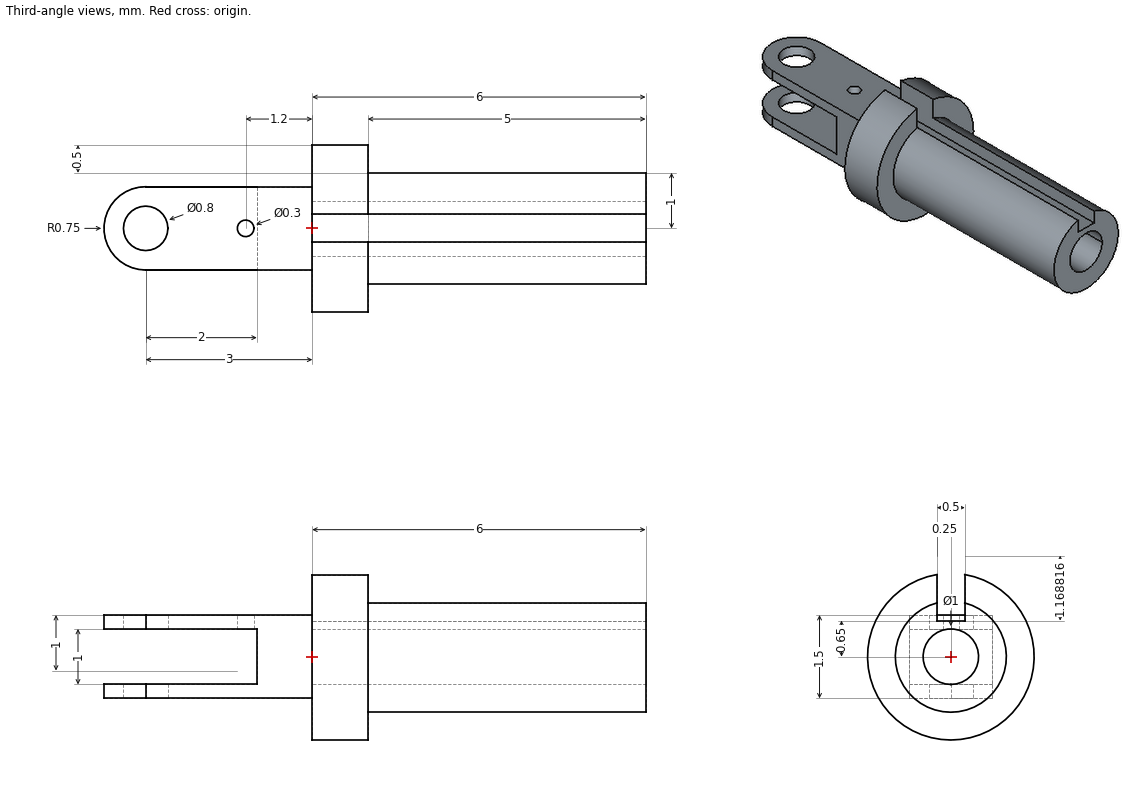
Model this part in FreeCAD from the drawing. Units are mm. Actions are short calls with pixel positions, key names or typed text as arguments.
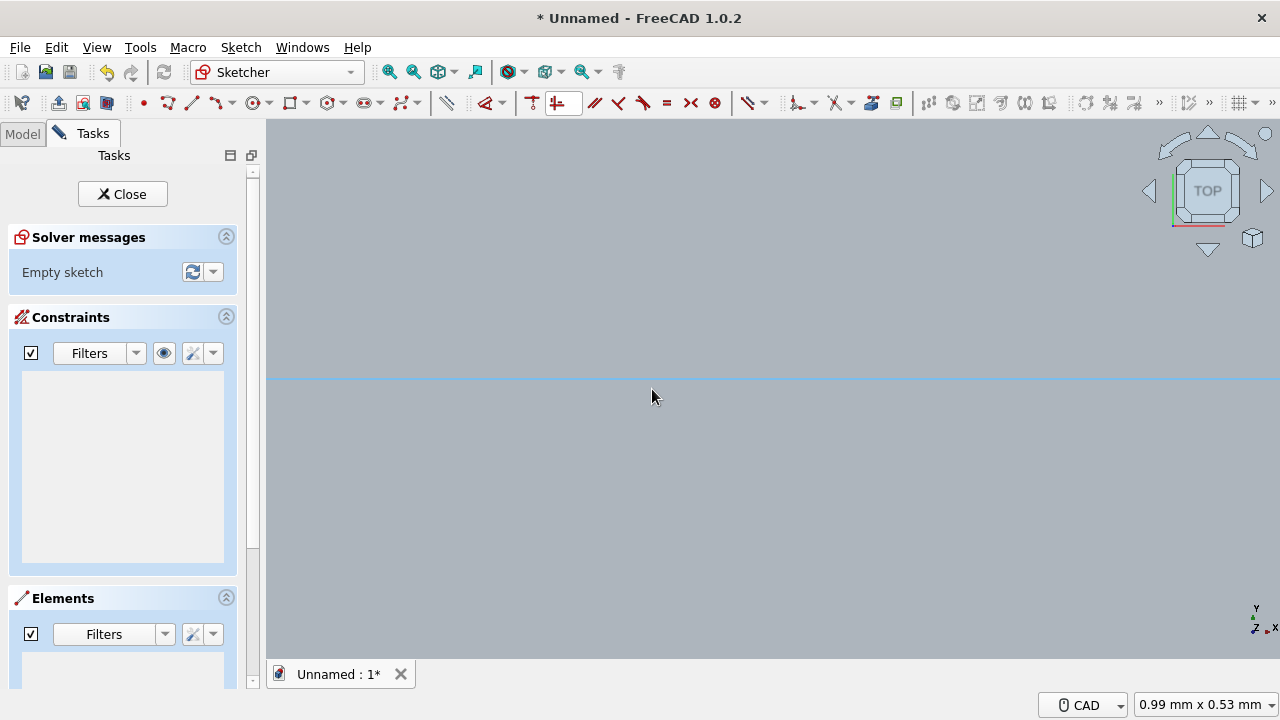
click(254, 104)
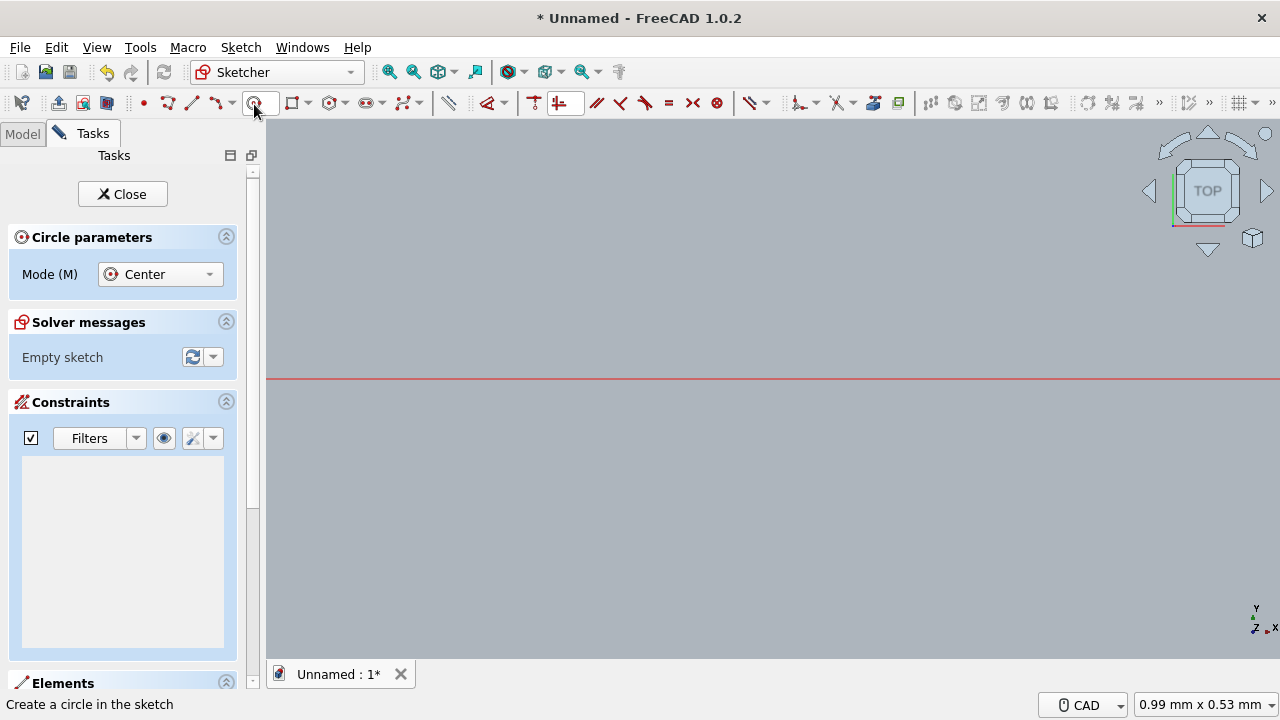
click(703, 379)
click(811, 271)
key(Escape)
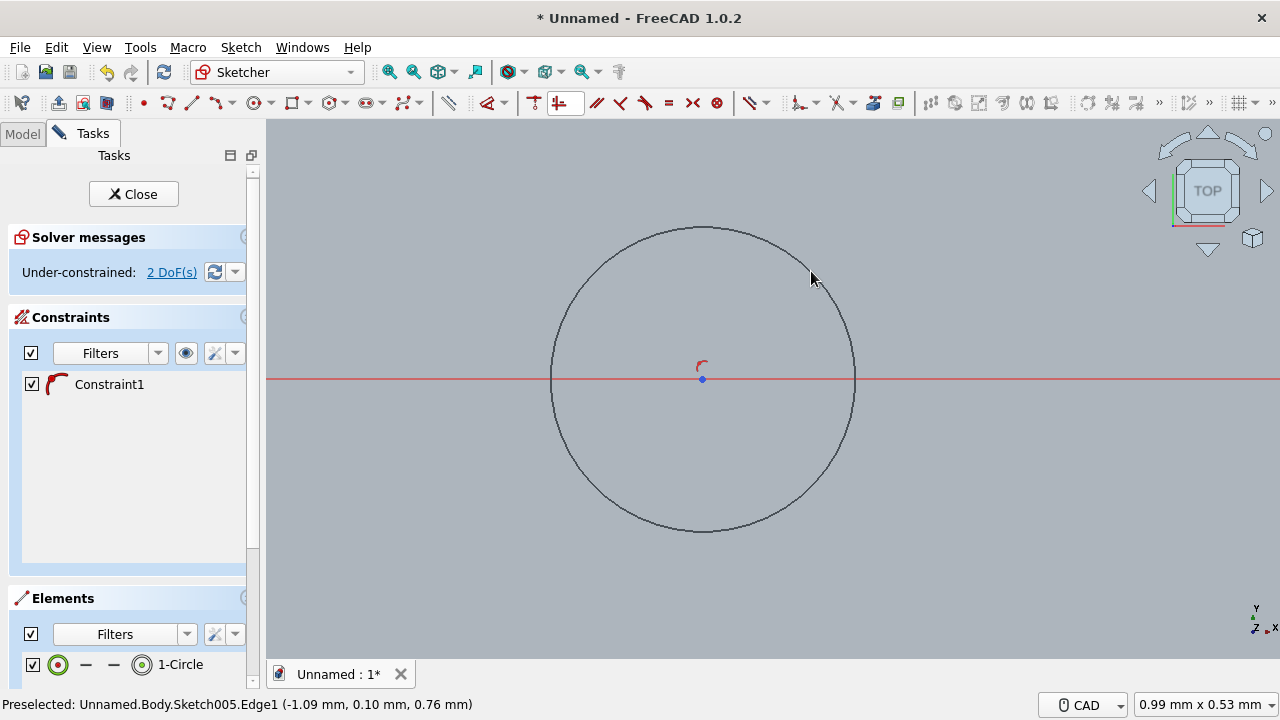
click(488, 104)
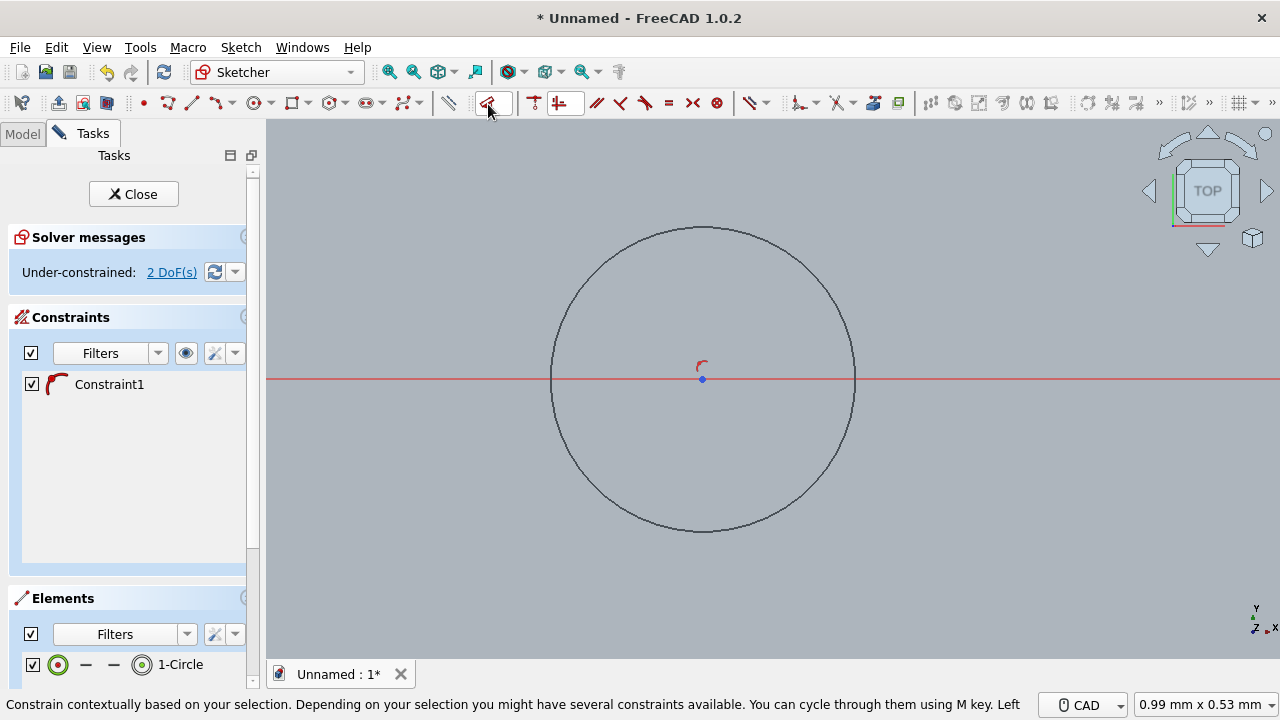
click(810, 271)
click(832, 248)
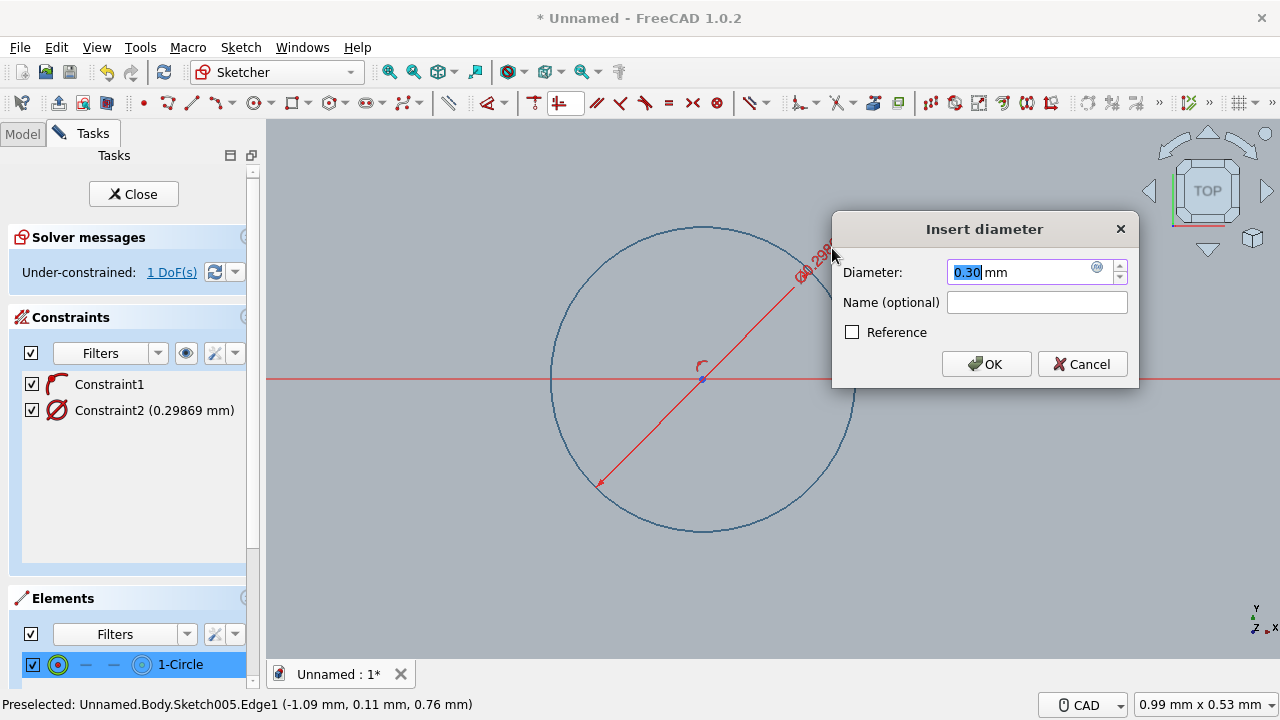
text(0.3)
key(Return)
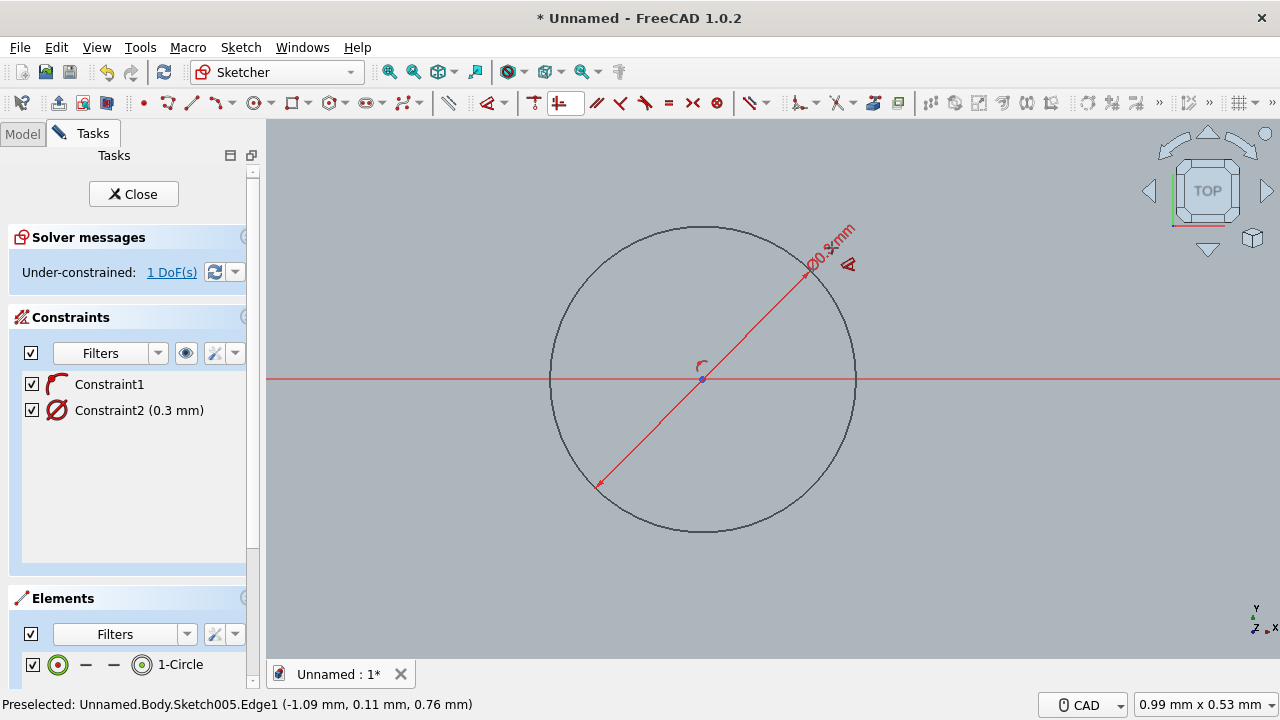
click(703, 379)
click(909, 413)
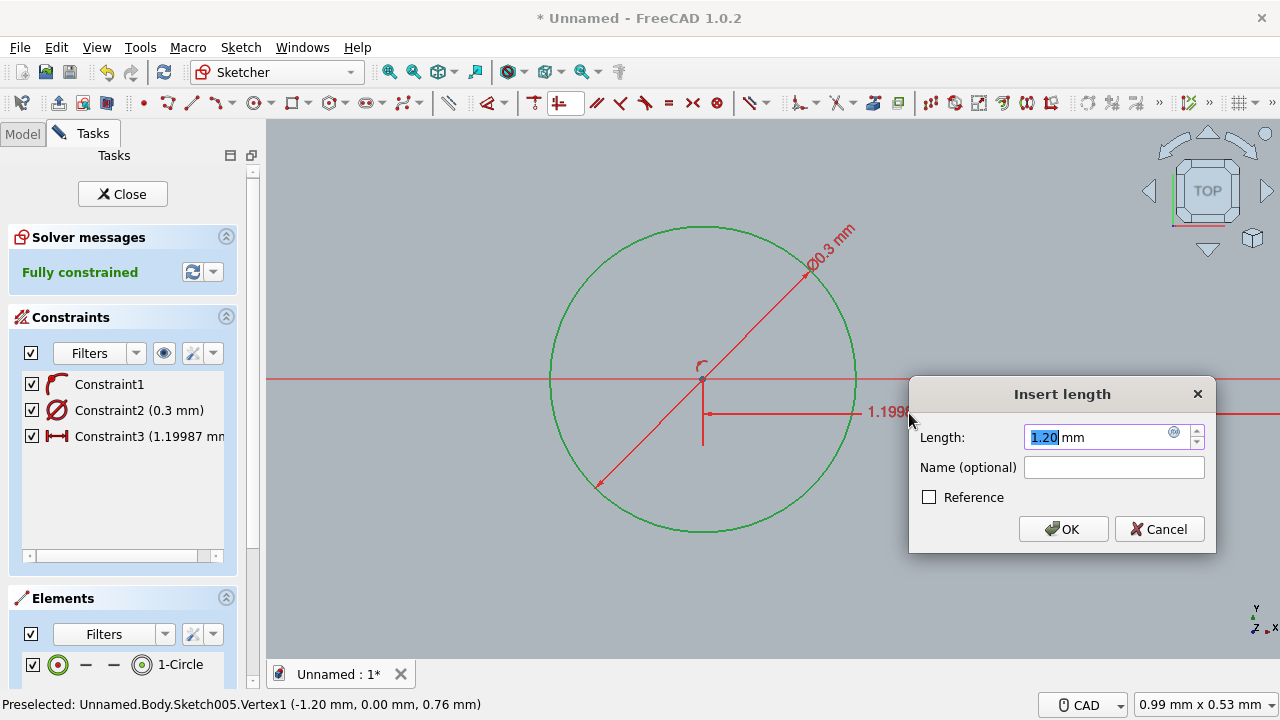
text(1.2)
key(Return)
key(Escape)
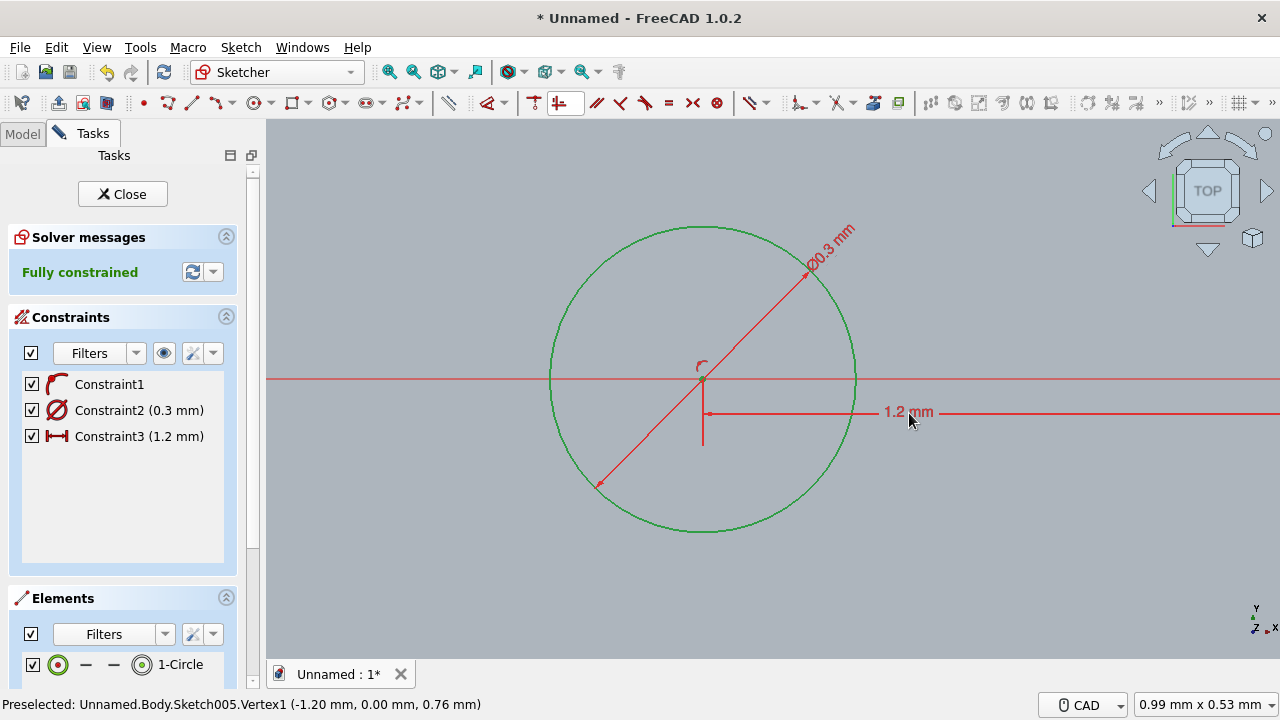
click(123, 194)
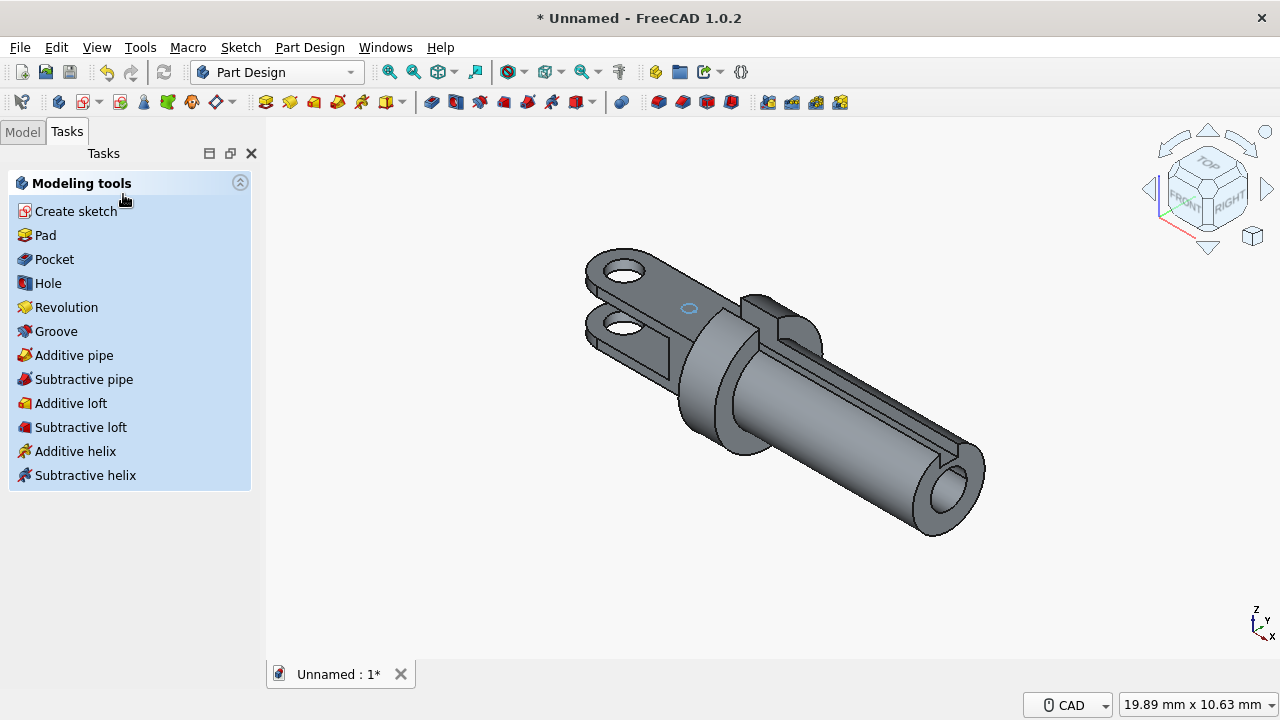
click(432, 102)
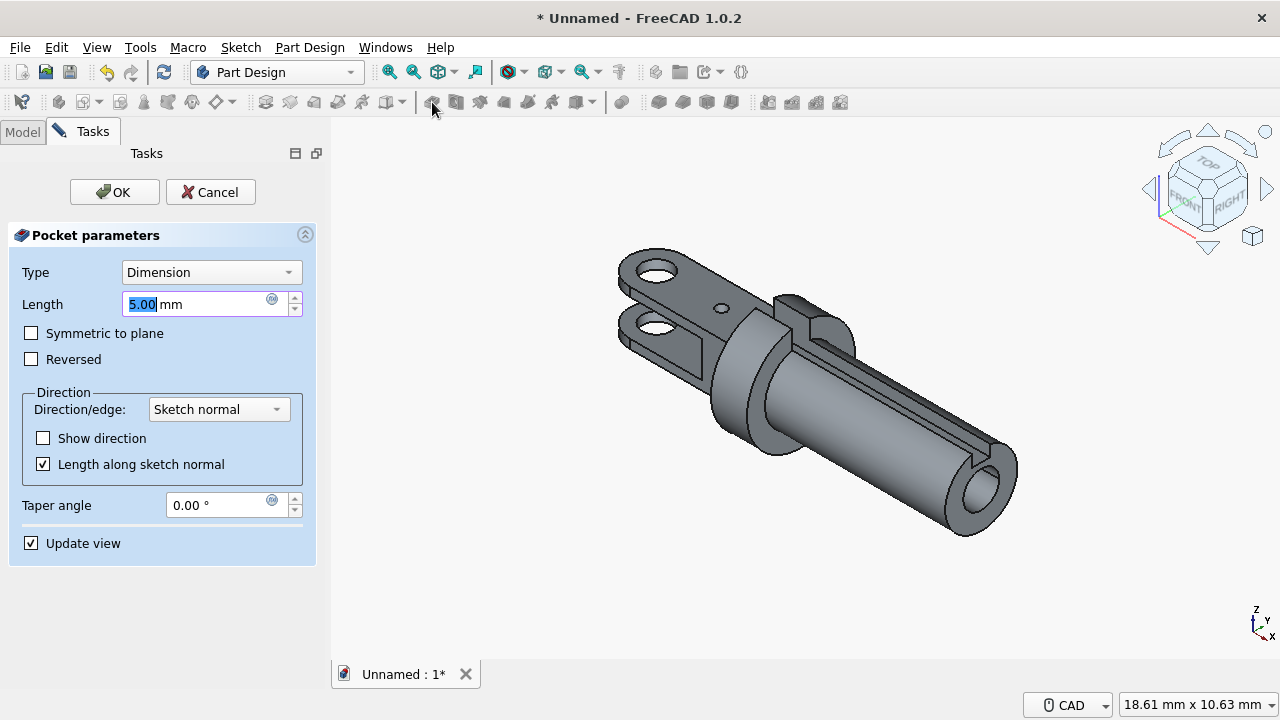
text(1)
key(Tab)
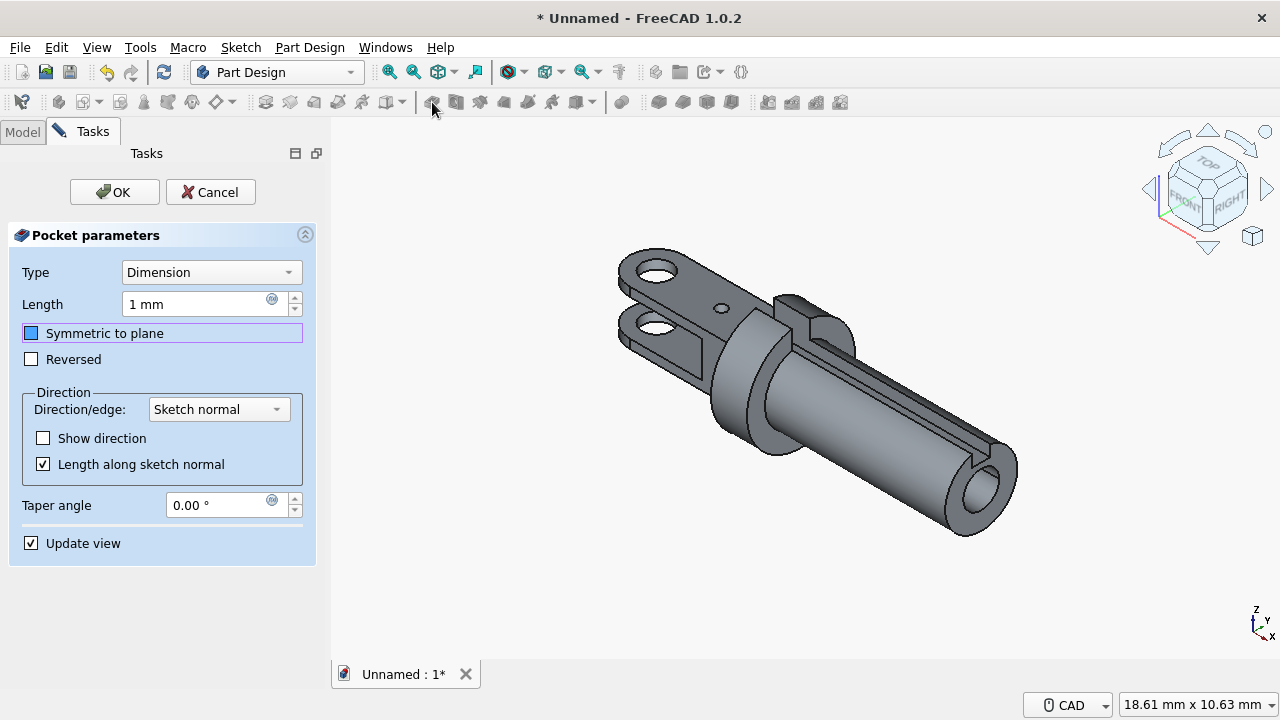
click(115, 192)